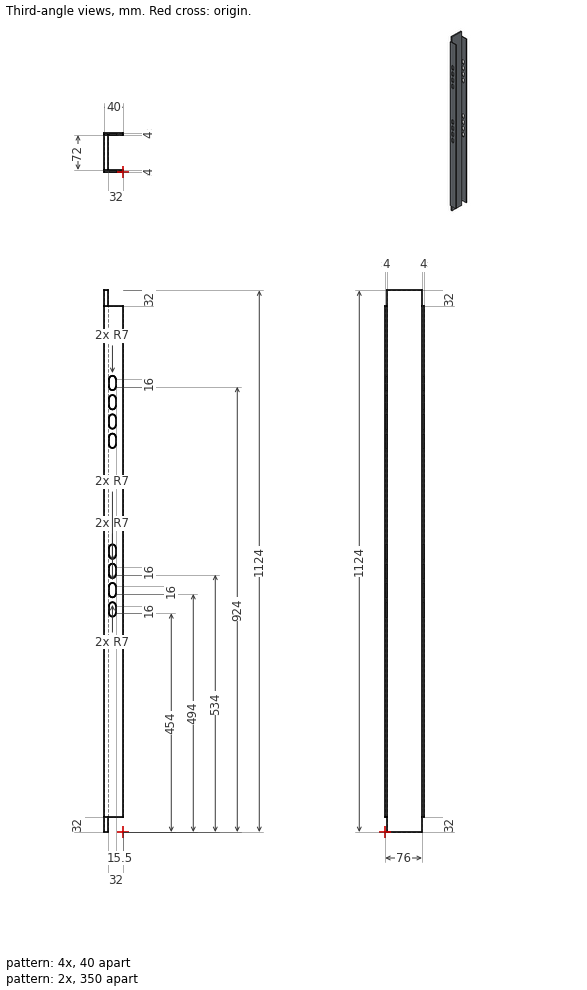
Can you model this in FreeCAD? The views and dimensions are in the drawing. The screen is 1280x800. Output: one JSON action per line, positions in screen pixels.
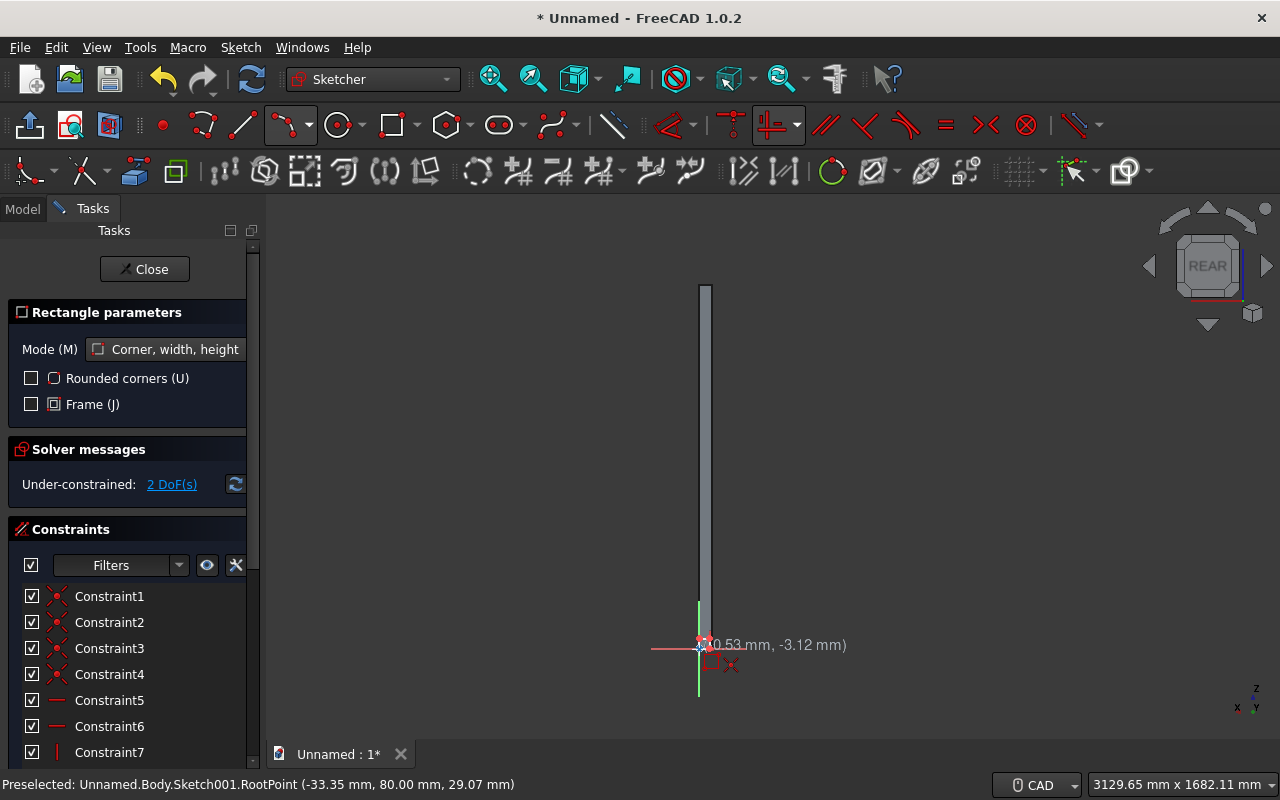
{"action": "scroll", "coordinate": [699, 285], "scroll_direction": "up", "scroll_amount": 3}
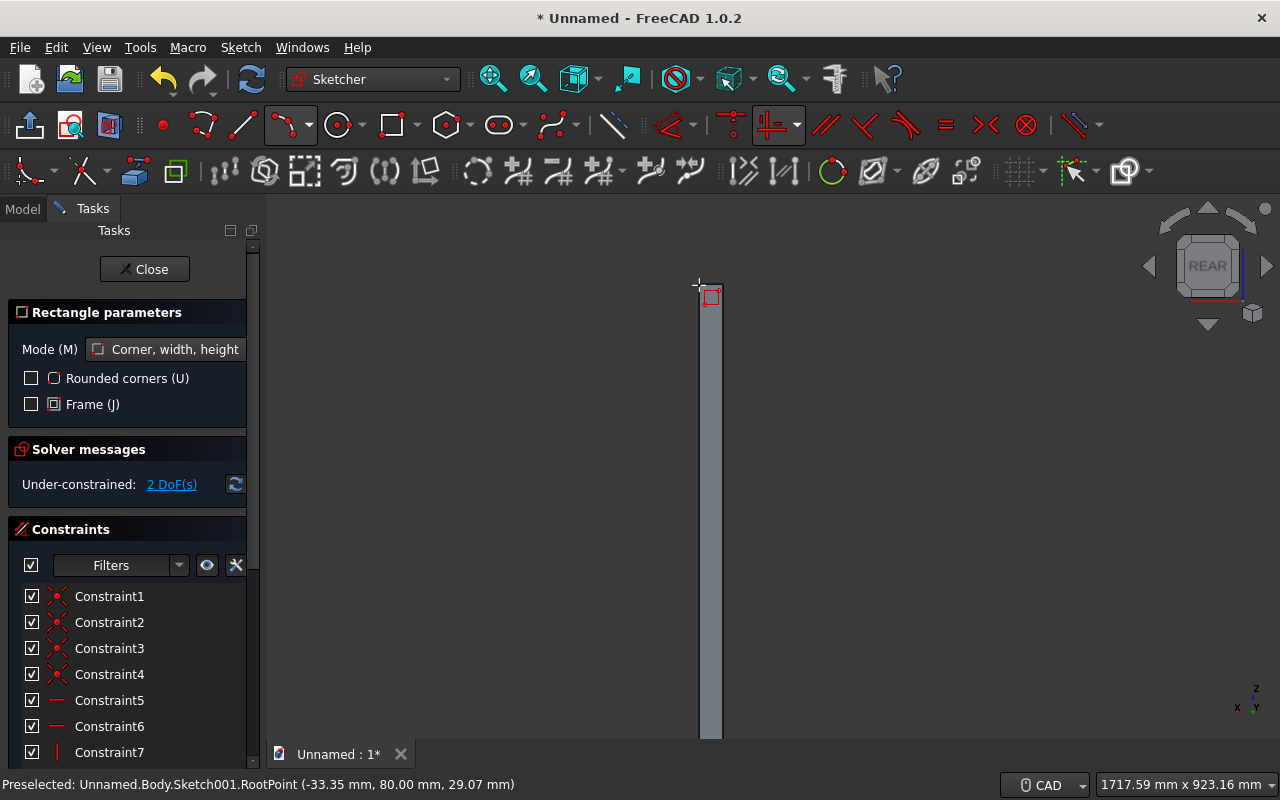
{"action": "left_click", "coordinate": [699, 284]}
{"action": "left_click", "coordinate": [718, 303]}
{"action": "key", "text": "Escape"}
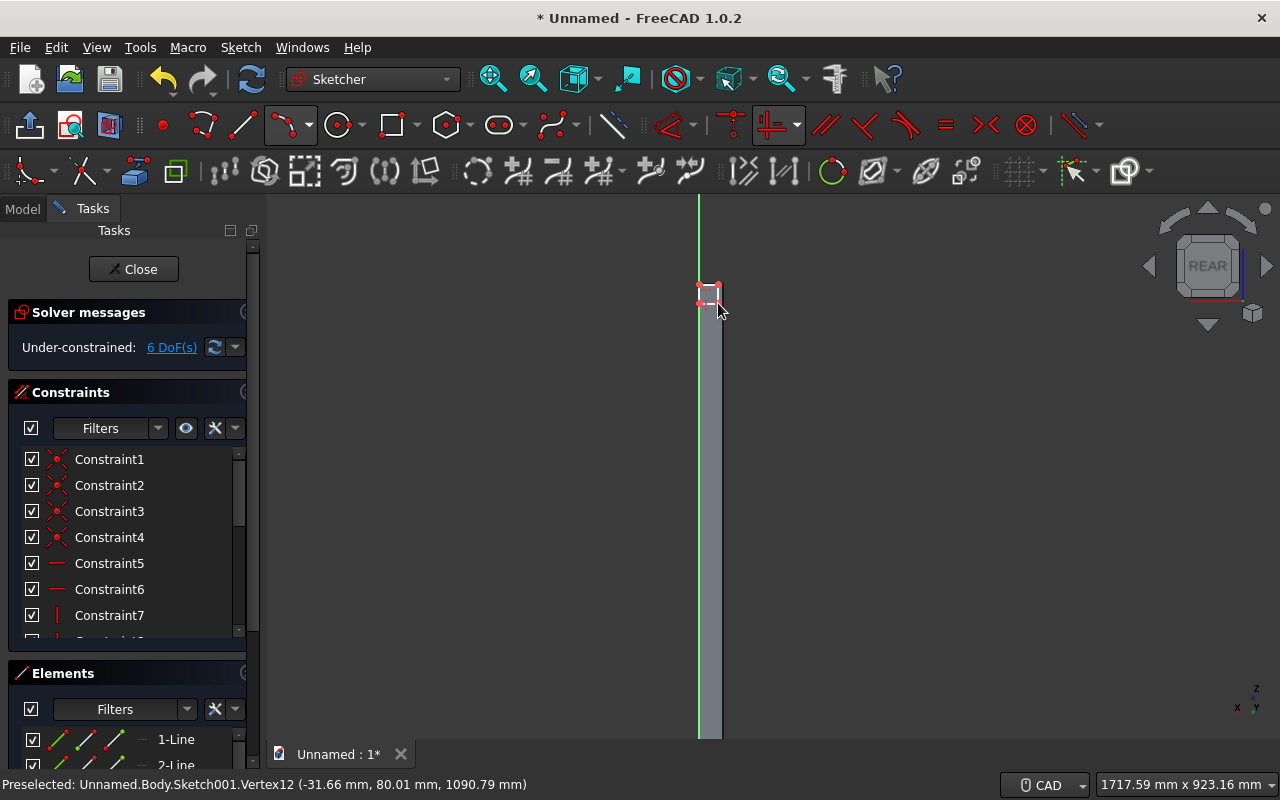
{"action": "left_click", "coordinate": [699, 285]}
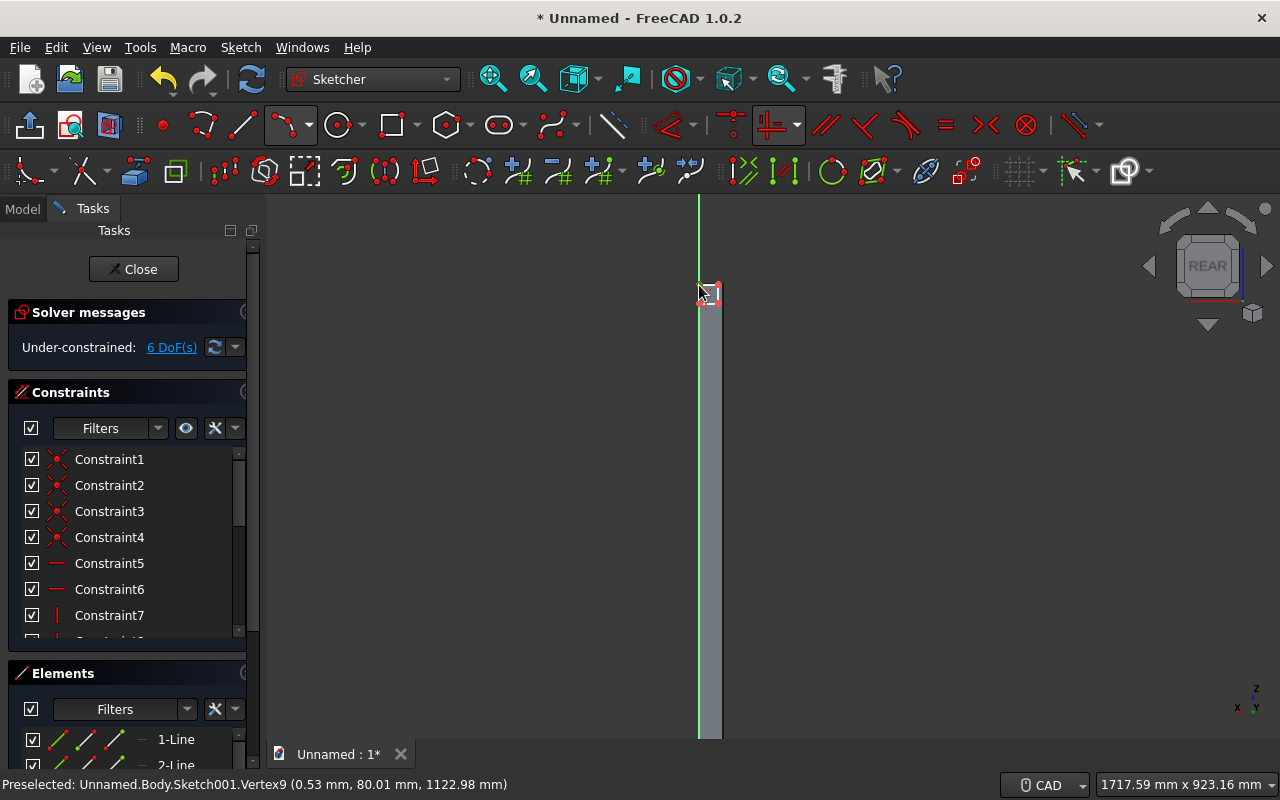
{"action": "left_click", "coordinate": [699, 676]}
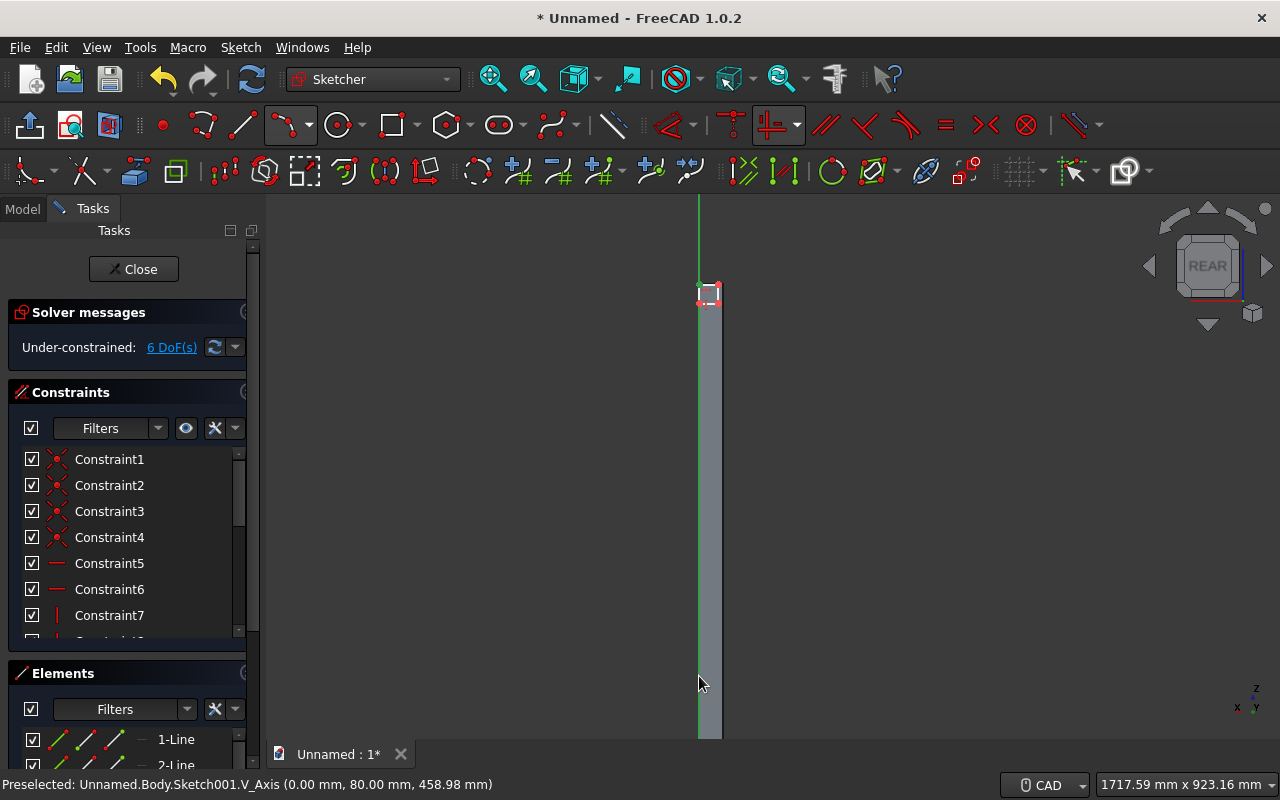
{"action": "left_click", "coordinate": [732, 126]}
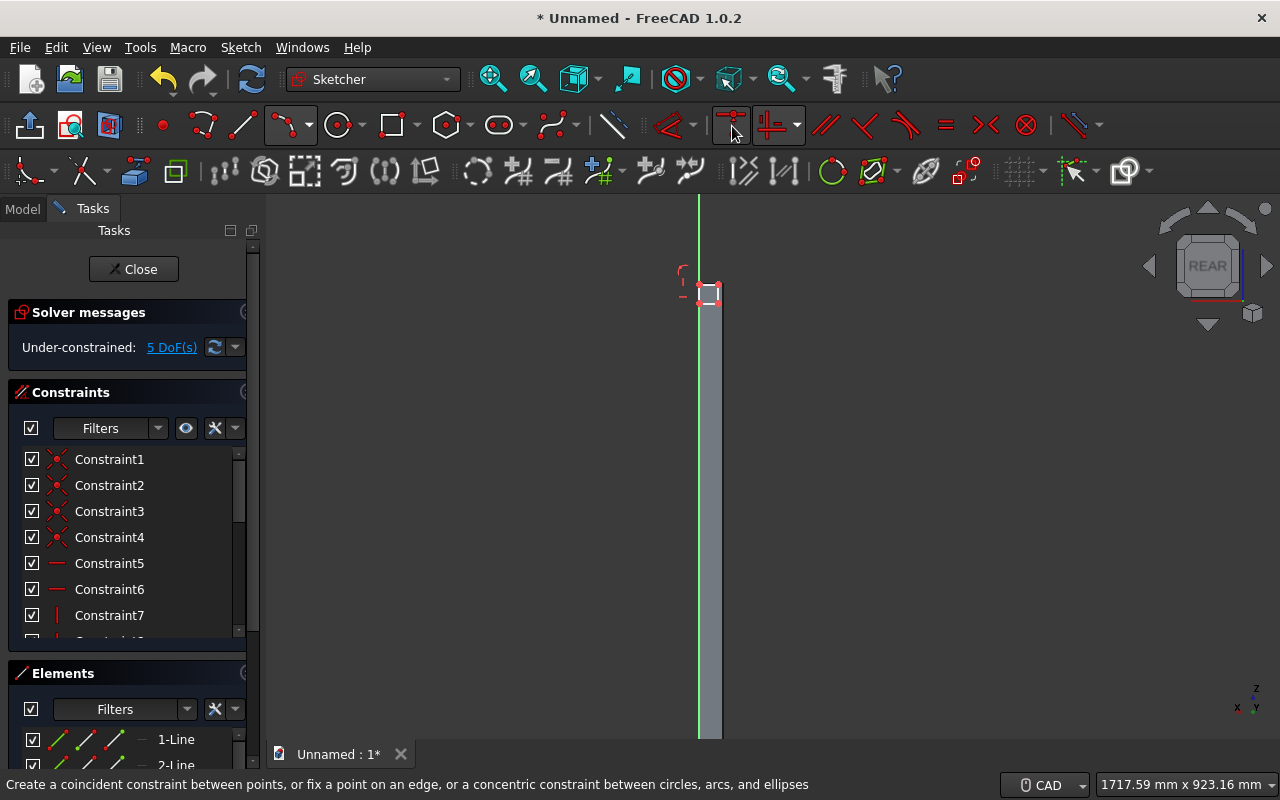
{"action": "left_click", "coordinate": [668, 126]}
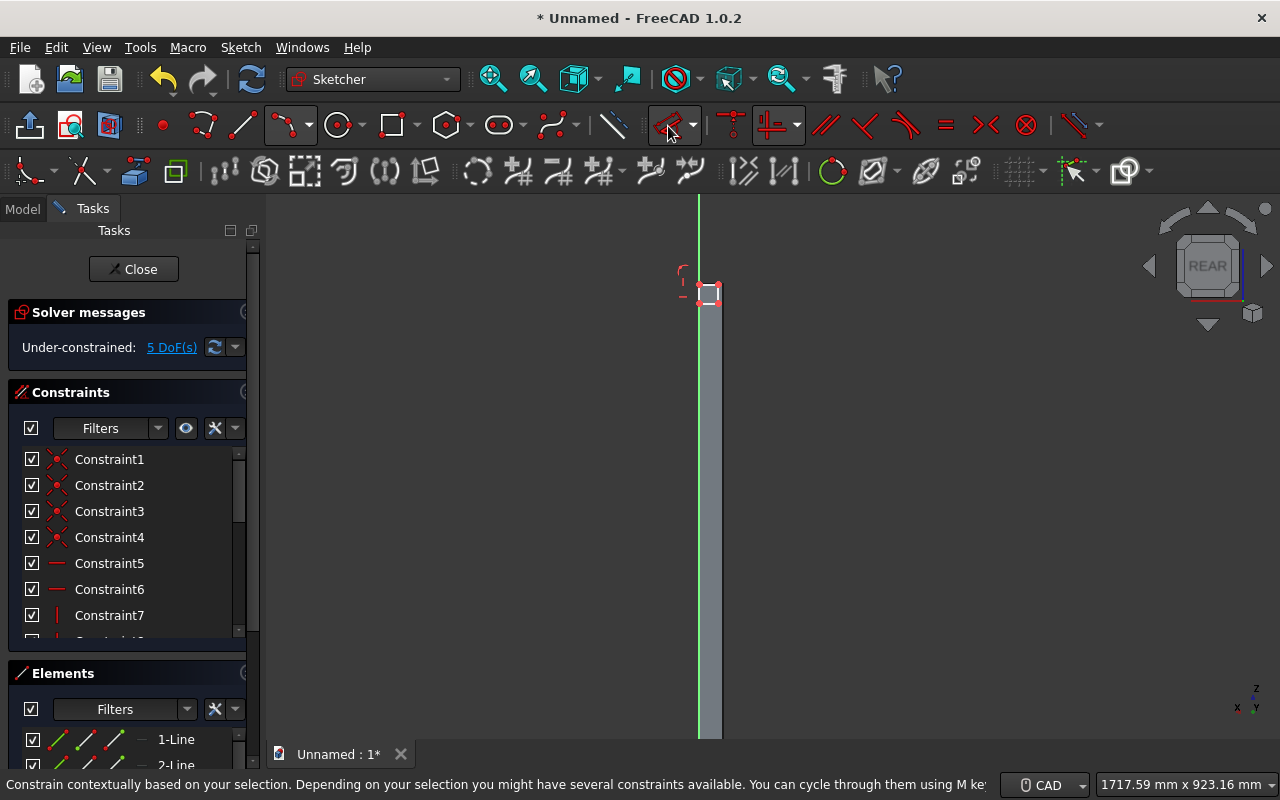
{"action": "scroll", "coordinate": [699, 284], "scroll_direction": "down", "scroll_amount": 3}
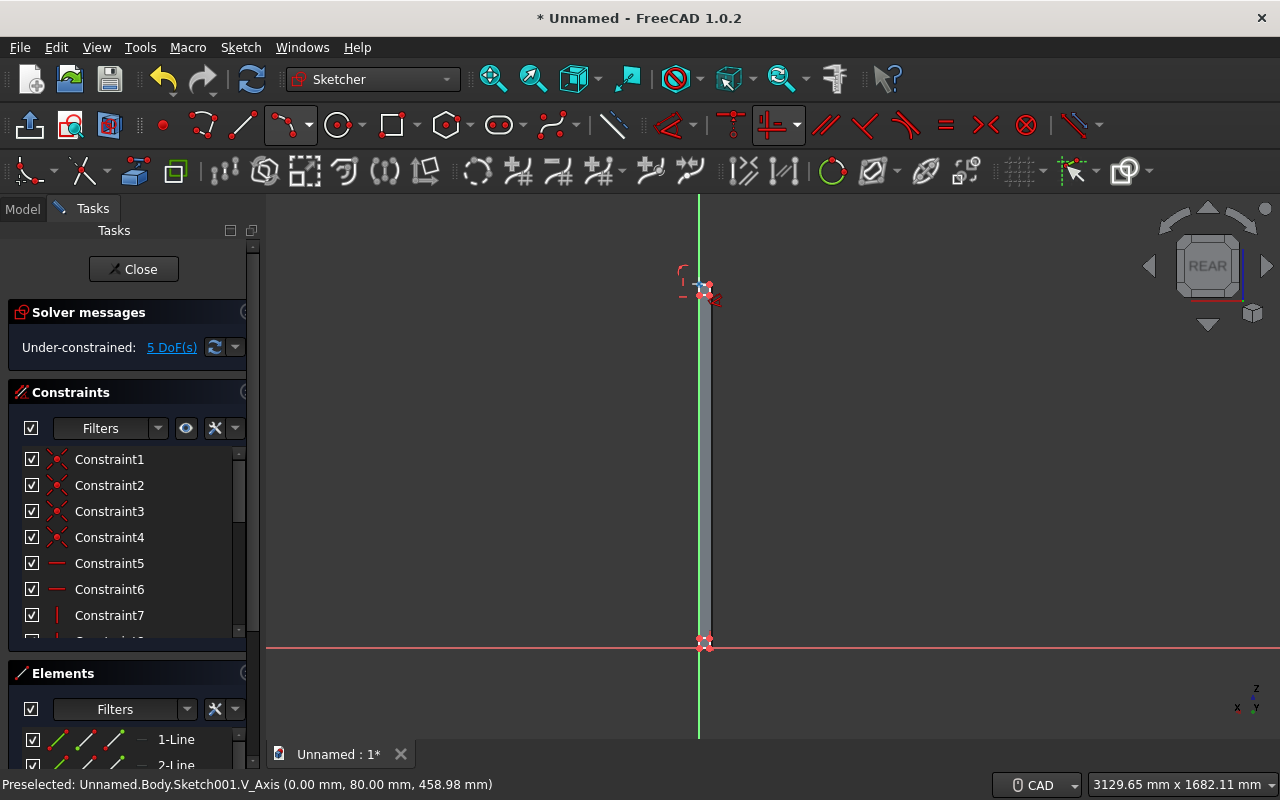
{"action": "scroll", "coordinate": [704, 648], "scroll_direction": "up", "scroll_amount": 7}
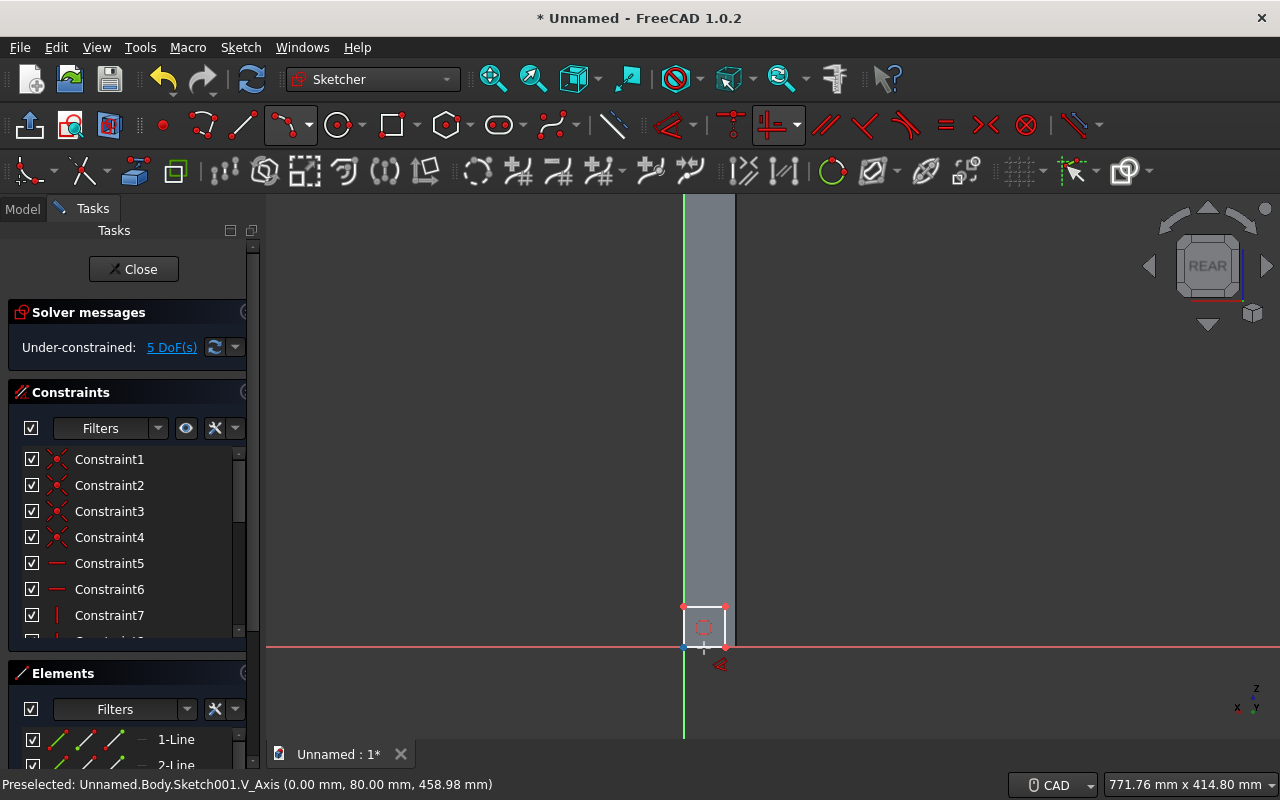
{"action": "left_click", "coordinate": [705, 647]}
{"action": "left_click", "coordinate": [705, 681]}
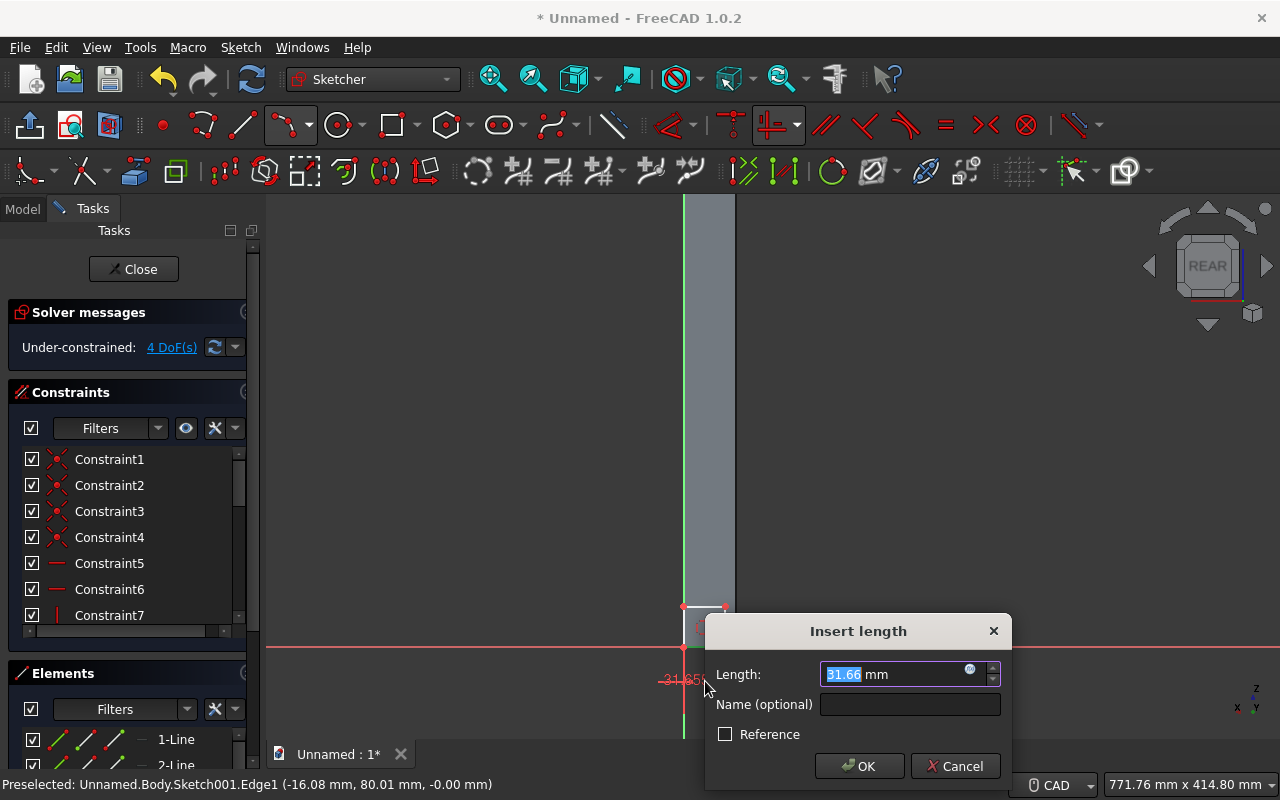
{"action": "type", "text": "32"}
{"action": "key", "text": "Return"}